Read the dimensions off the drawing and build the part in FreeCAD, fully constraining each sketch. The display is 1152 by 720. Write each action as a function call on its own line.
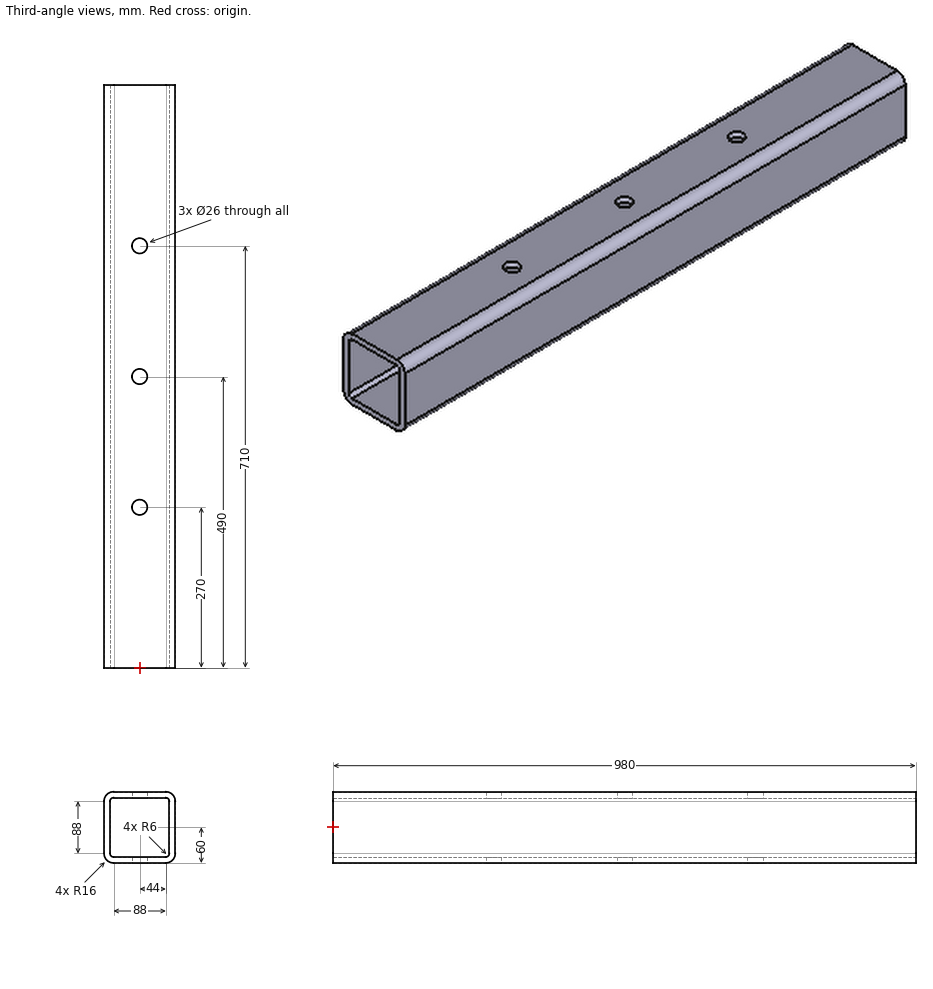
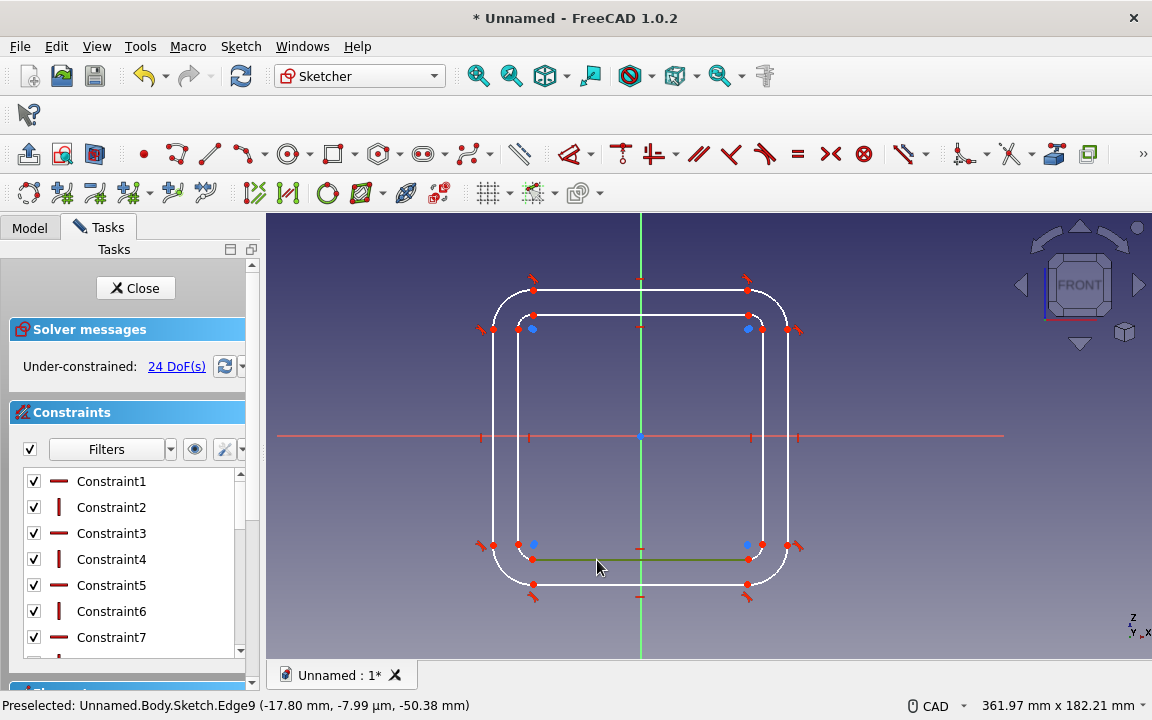
scroll(758, 555, up, 2)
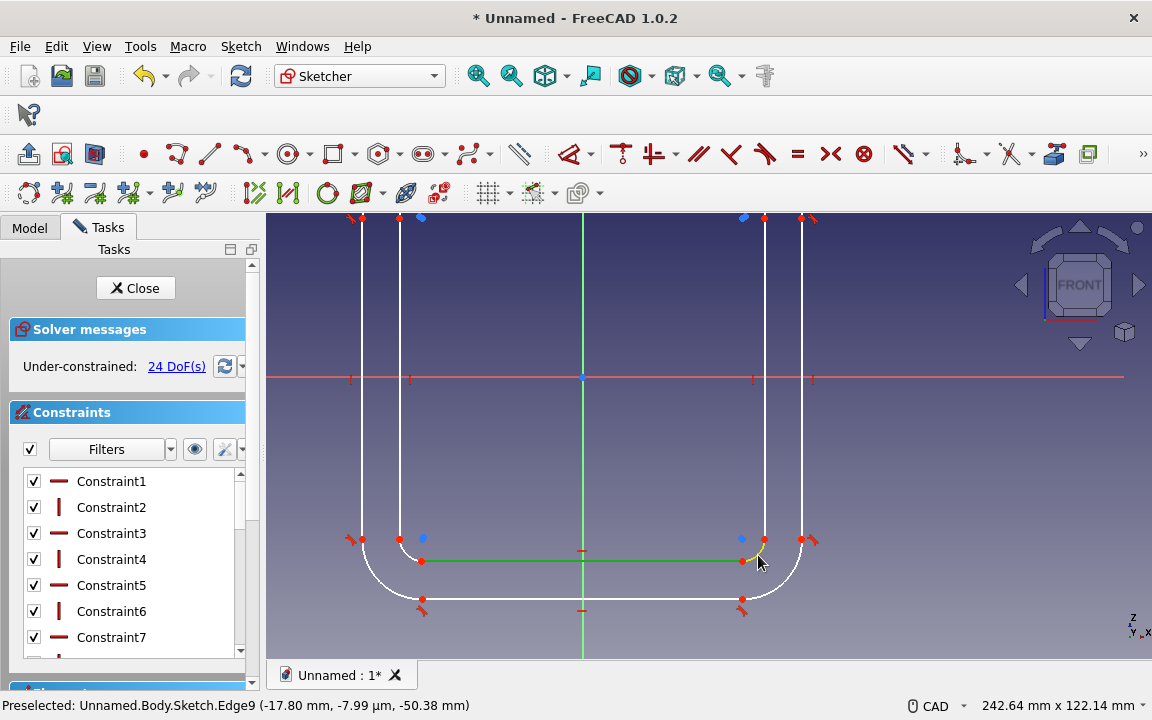
click(758, 555)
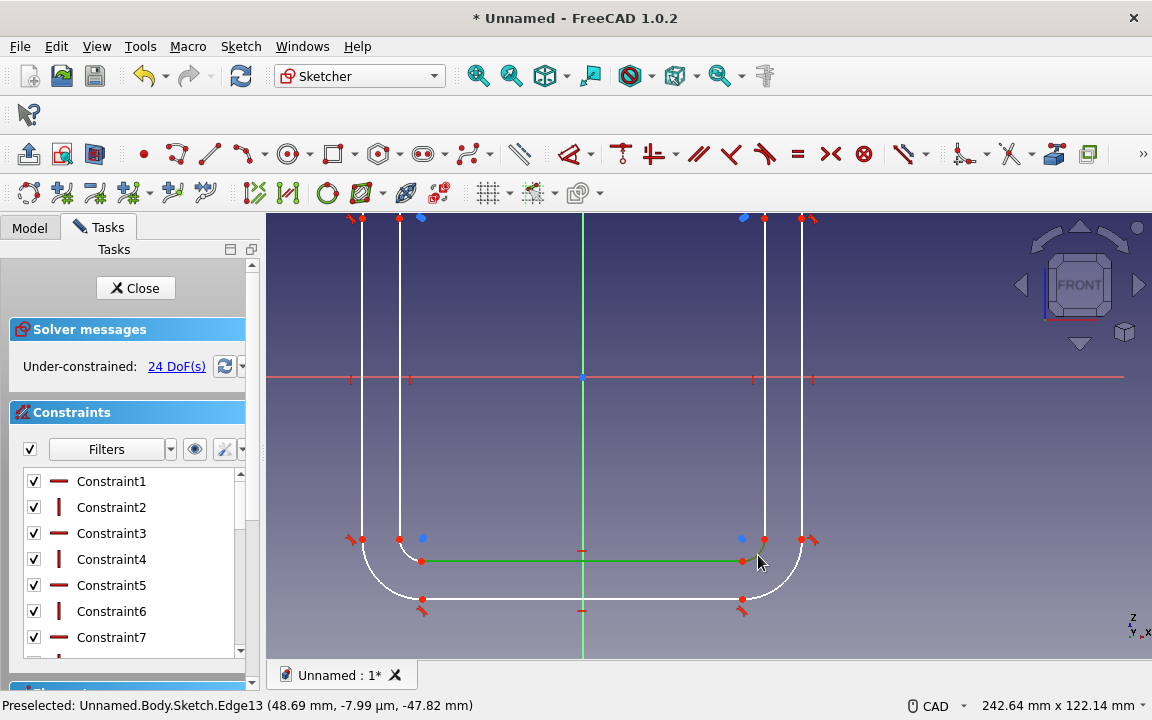
click(765, 154)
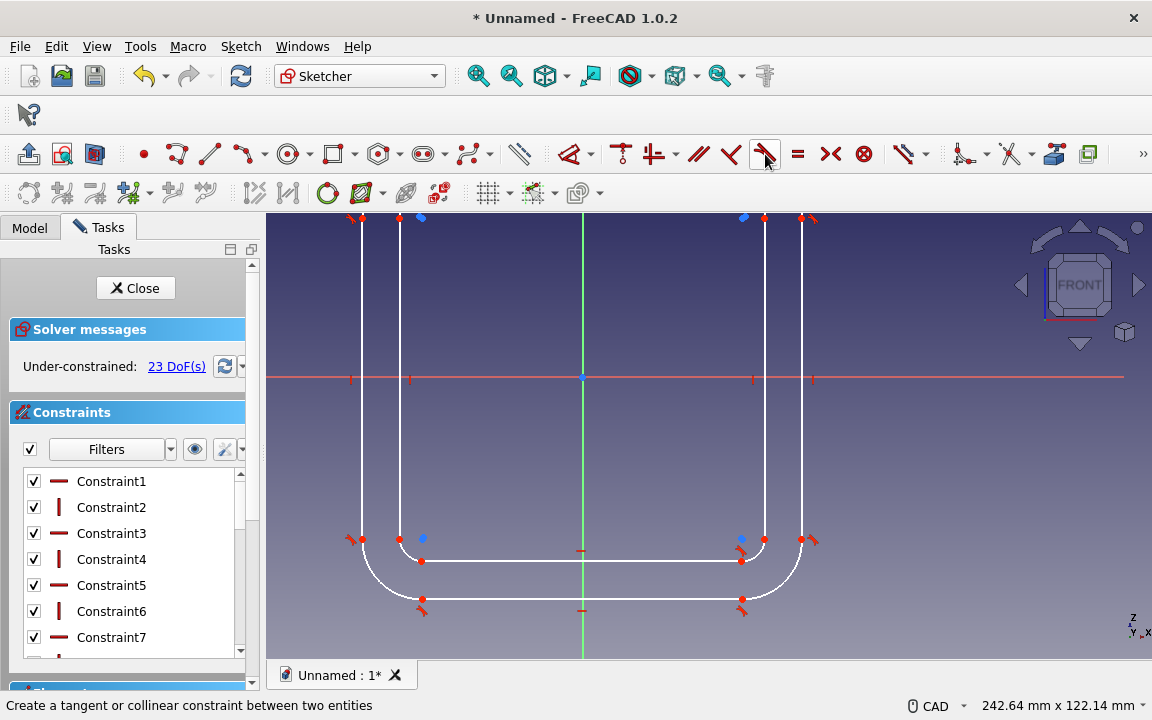
click(518, 561)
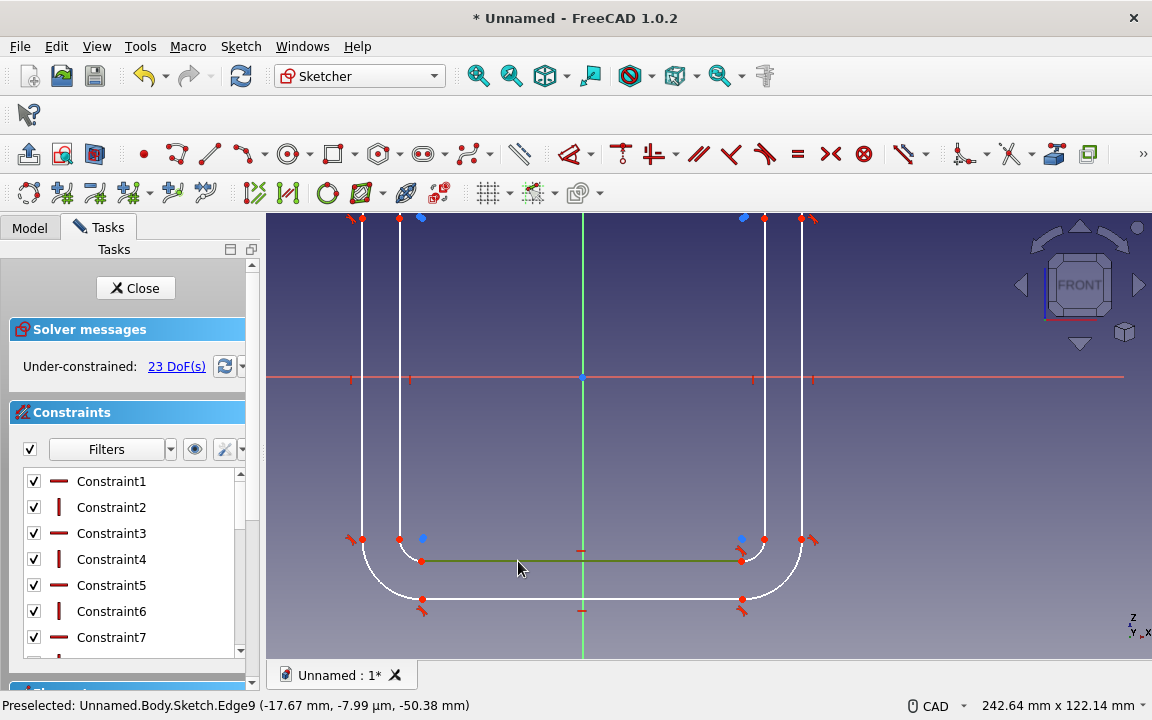
scroll(403, 549, up, 2)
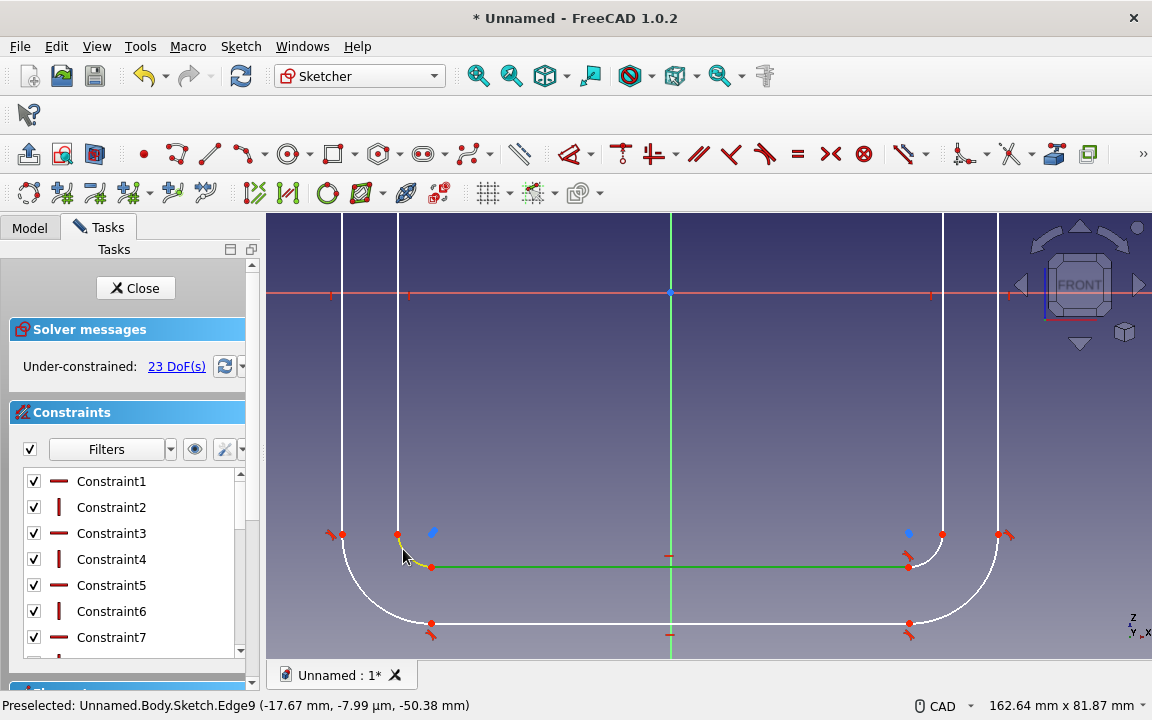
click(403, 549)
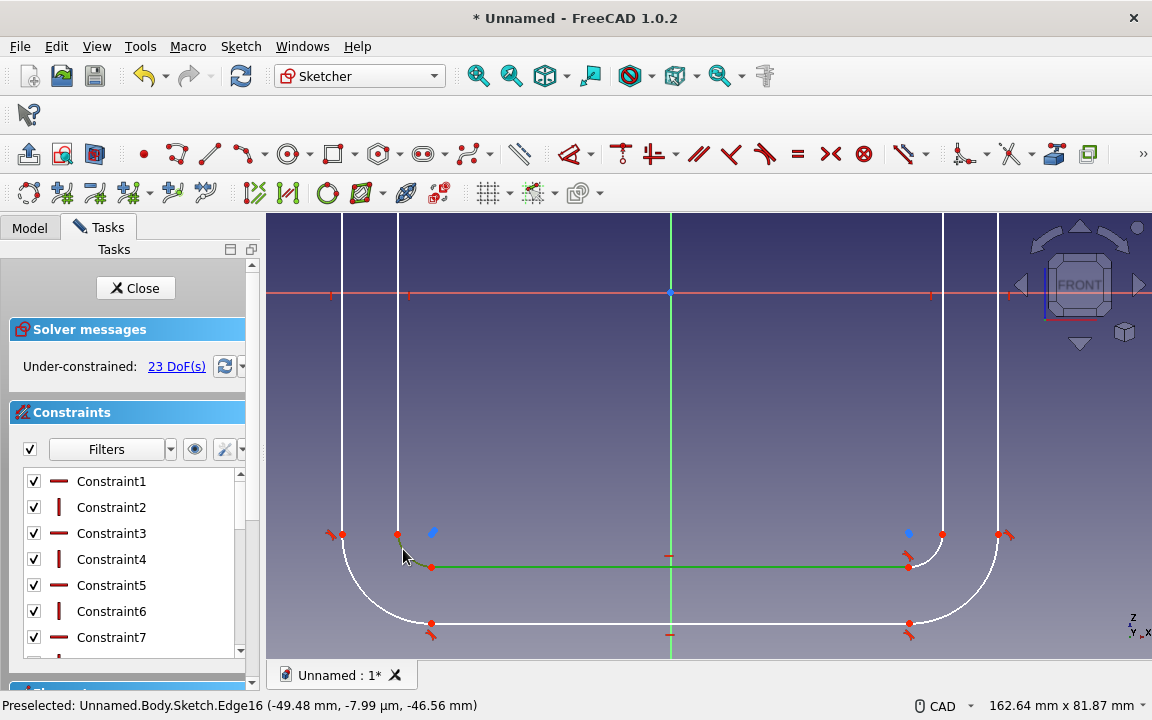
click(765, 154)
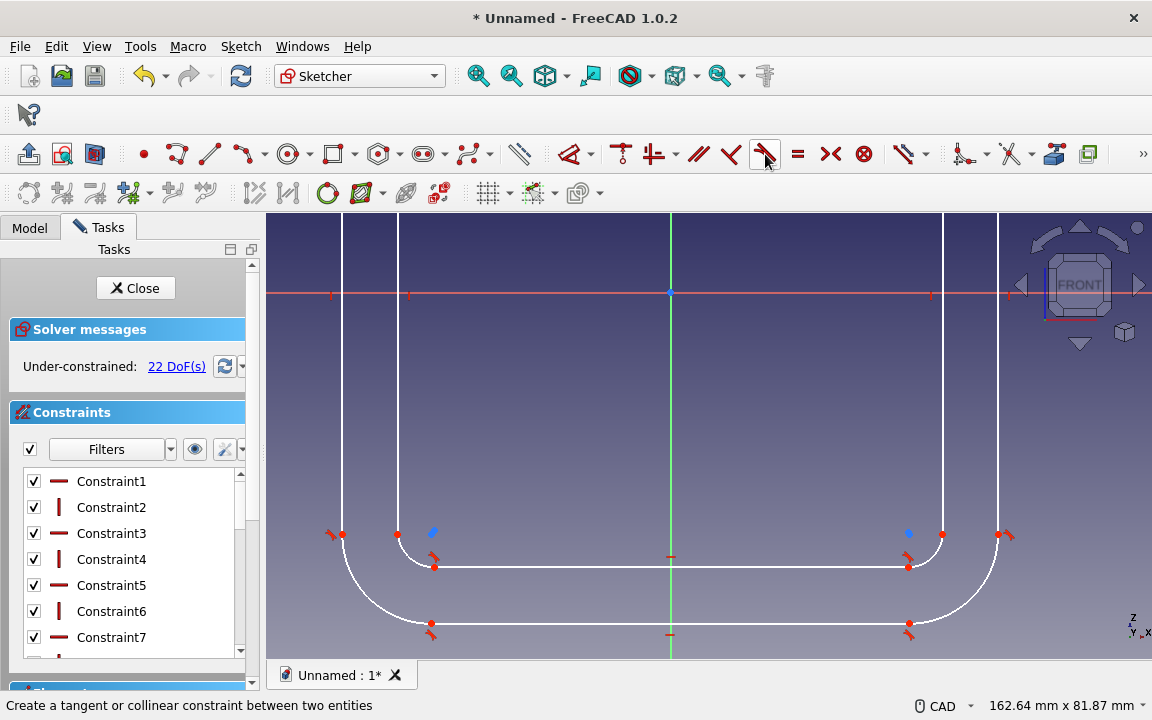
click(943, 391)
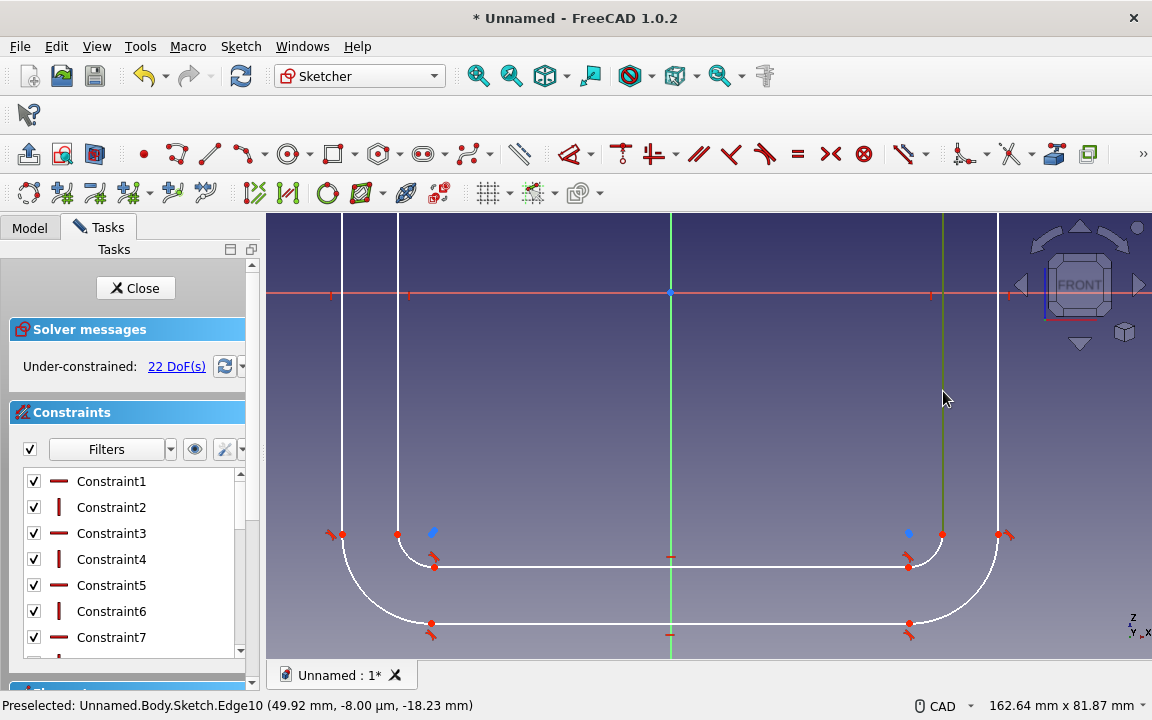
click(923, 564)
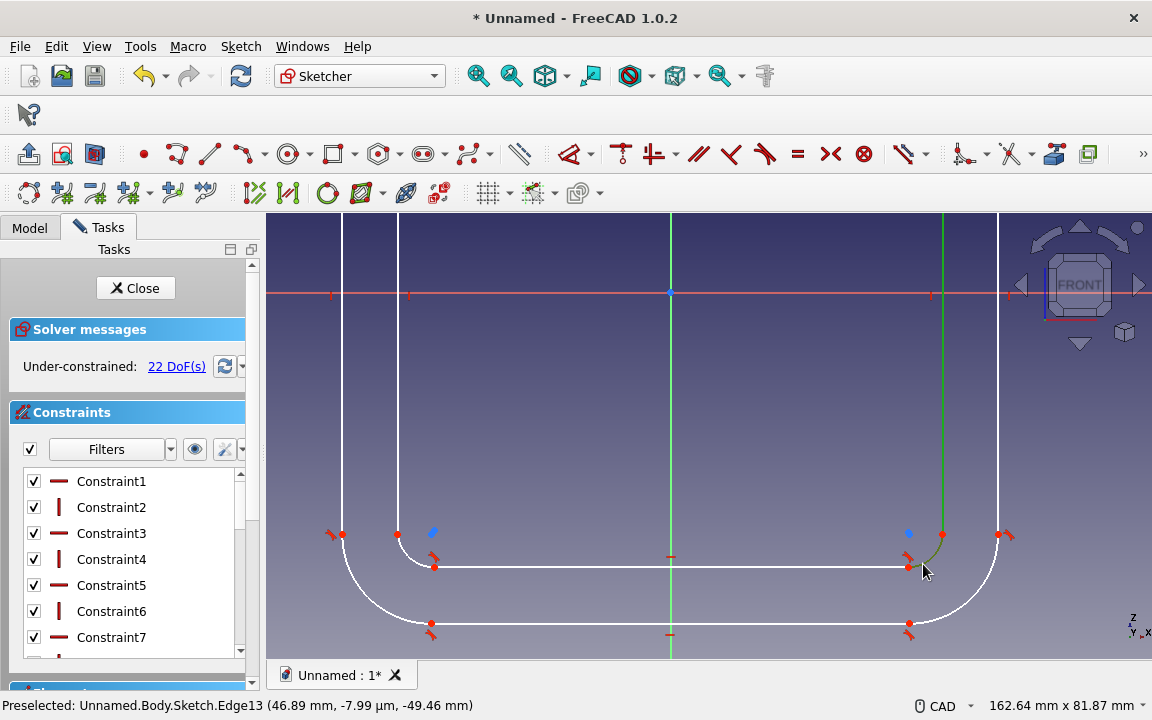
click(765, 154)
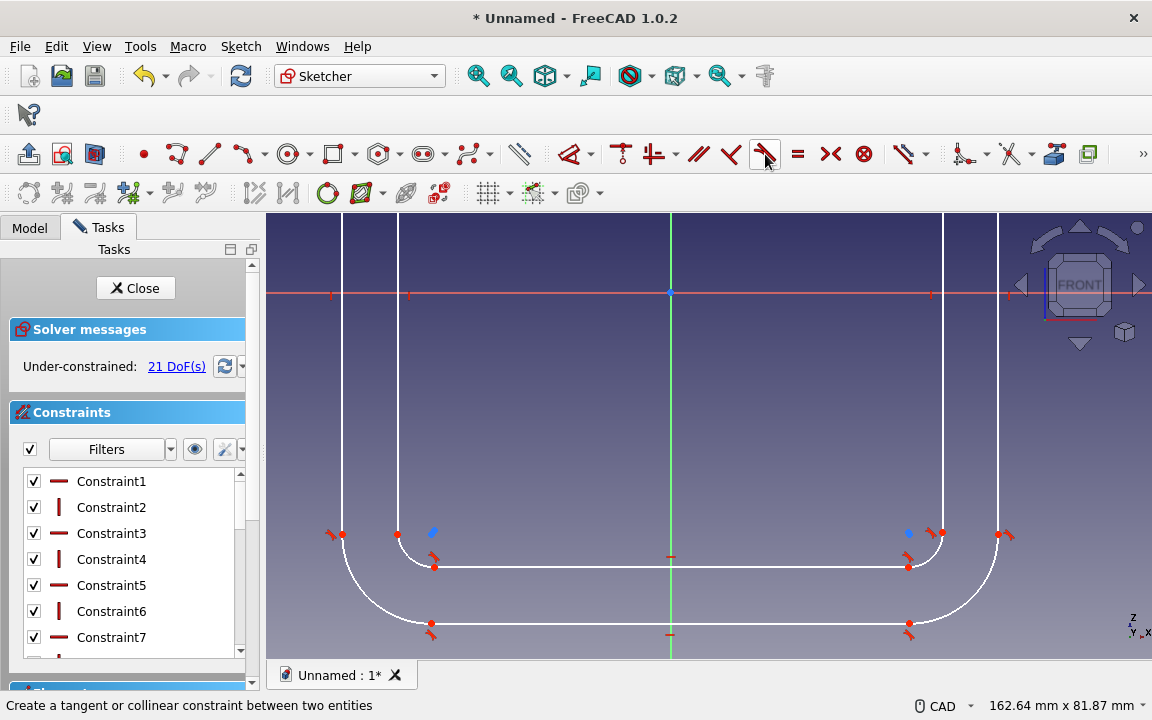
click(943, 390)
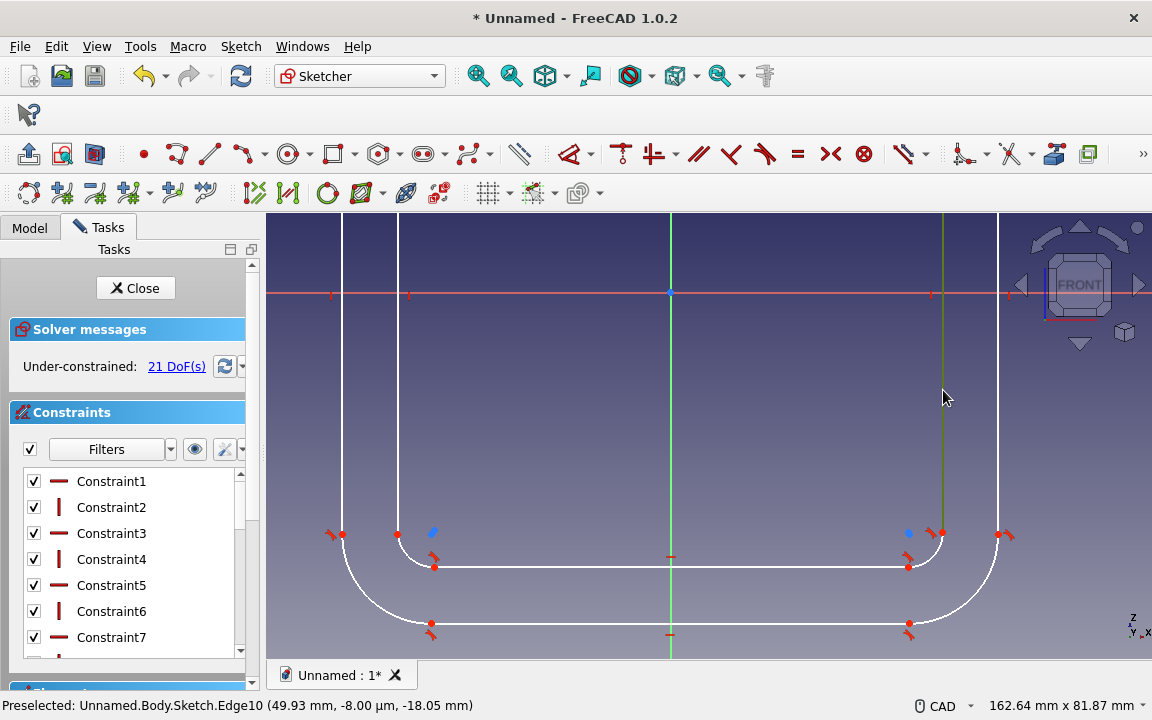
scroll(616, 553, down, 4)